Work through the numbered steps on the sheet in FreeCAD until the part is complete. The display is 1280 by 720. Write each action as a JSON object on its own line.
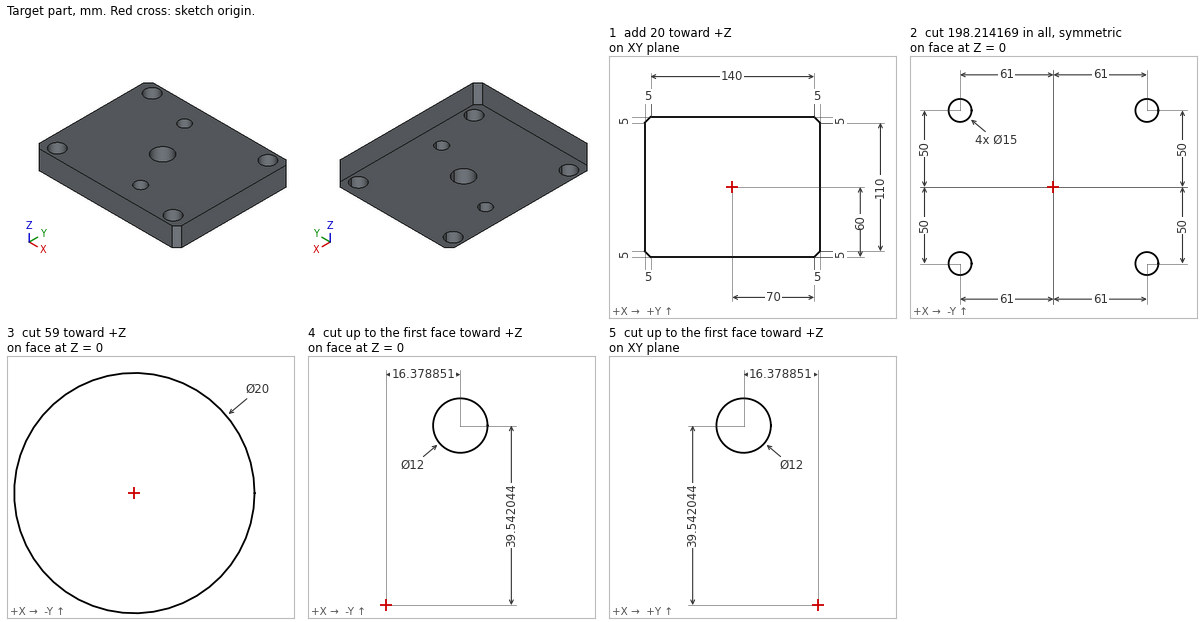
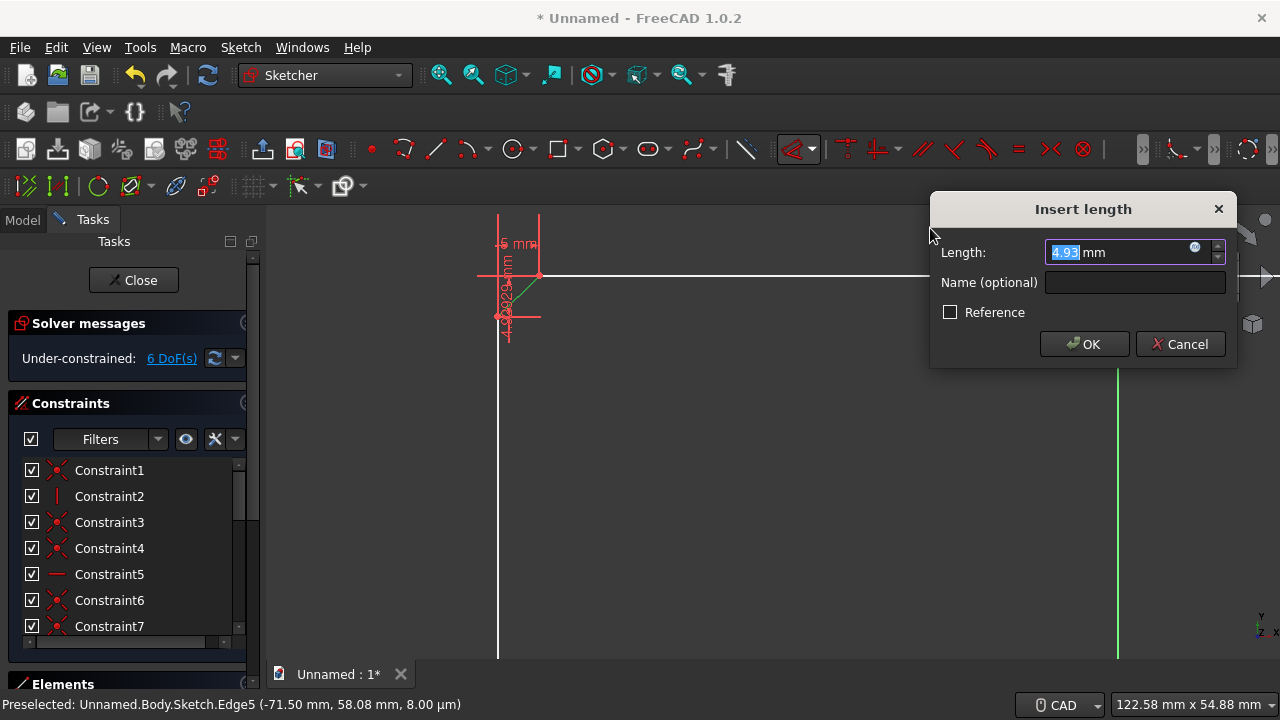
{"action": "type", "text": "5"}
{"action": "key", "text": "Return"}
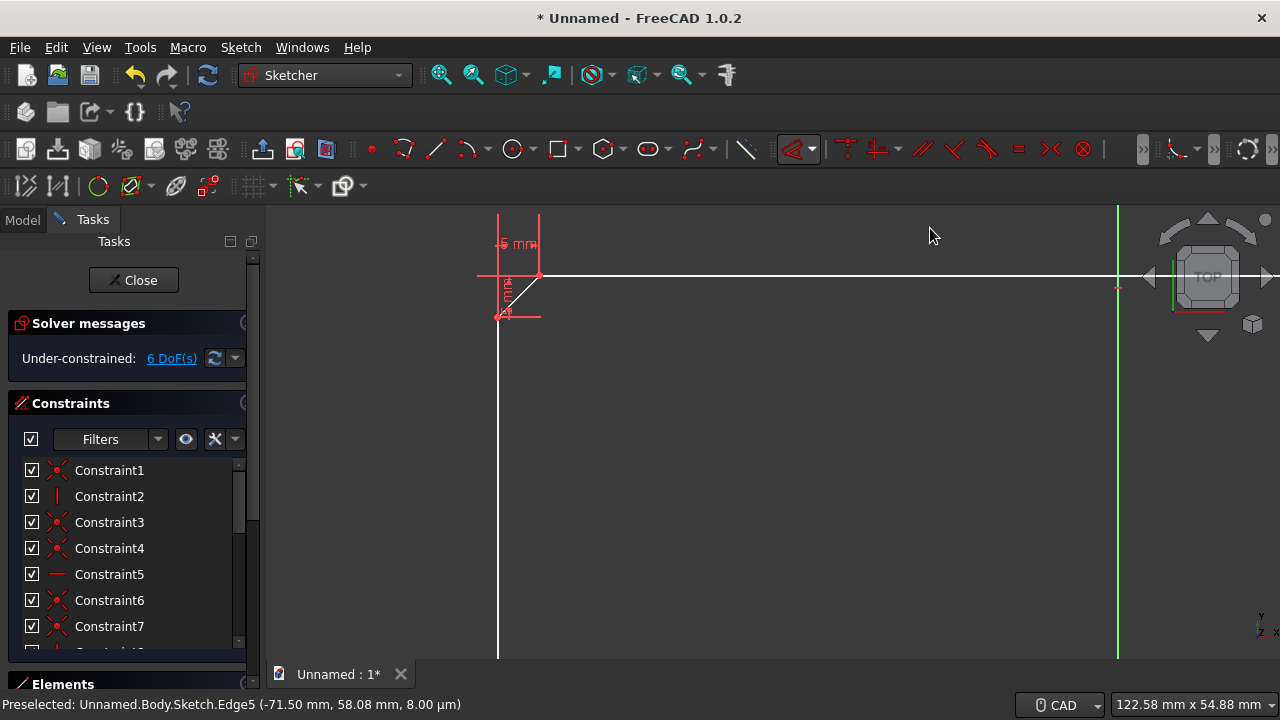
{"action": "scroll", "coordinate": [526, 287], "scroll_direction": "down", "scroll_amount": 6}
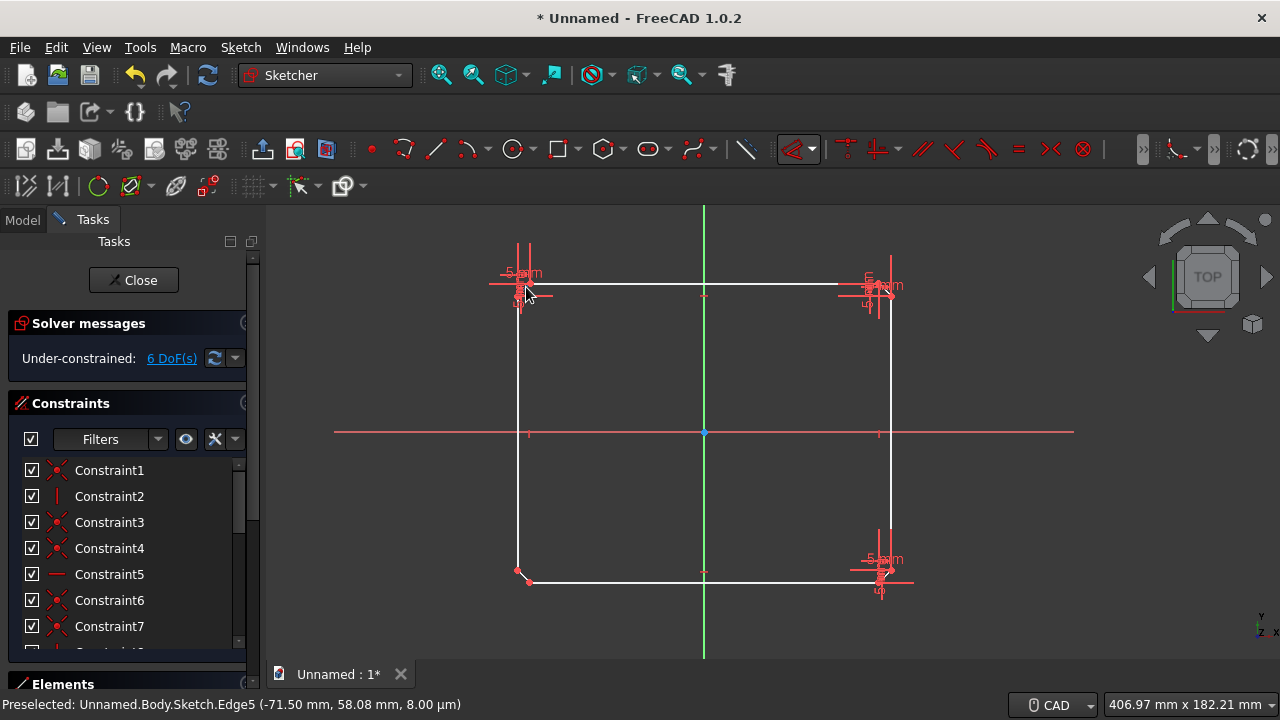
{"action": "scroll", "coordinate": [521, 574], "scroll_direction": "up", "scroll_amount": 6}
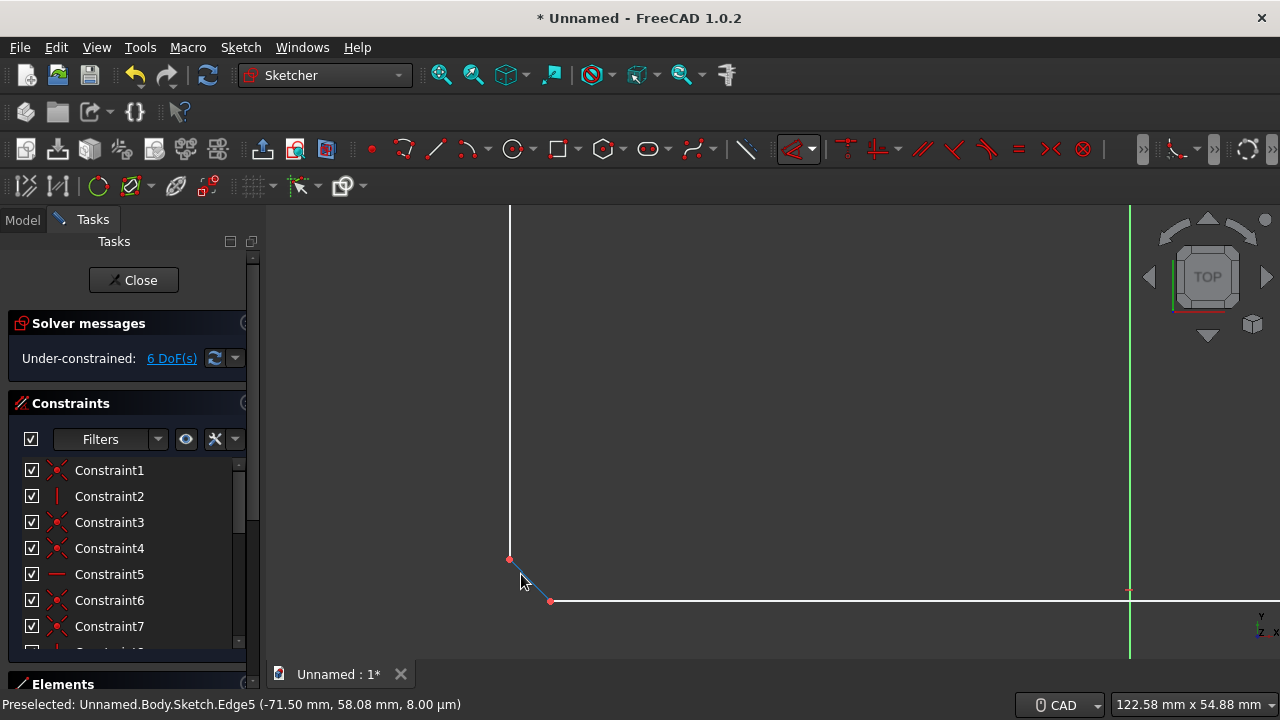
{"action": "left_click", "coordinate": [522, 572]}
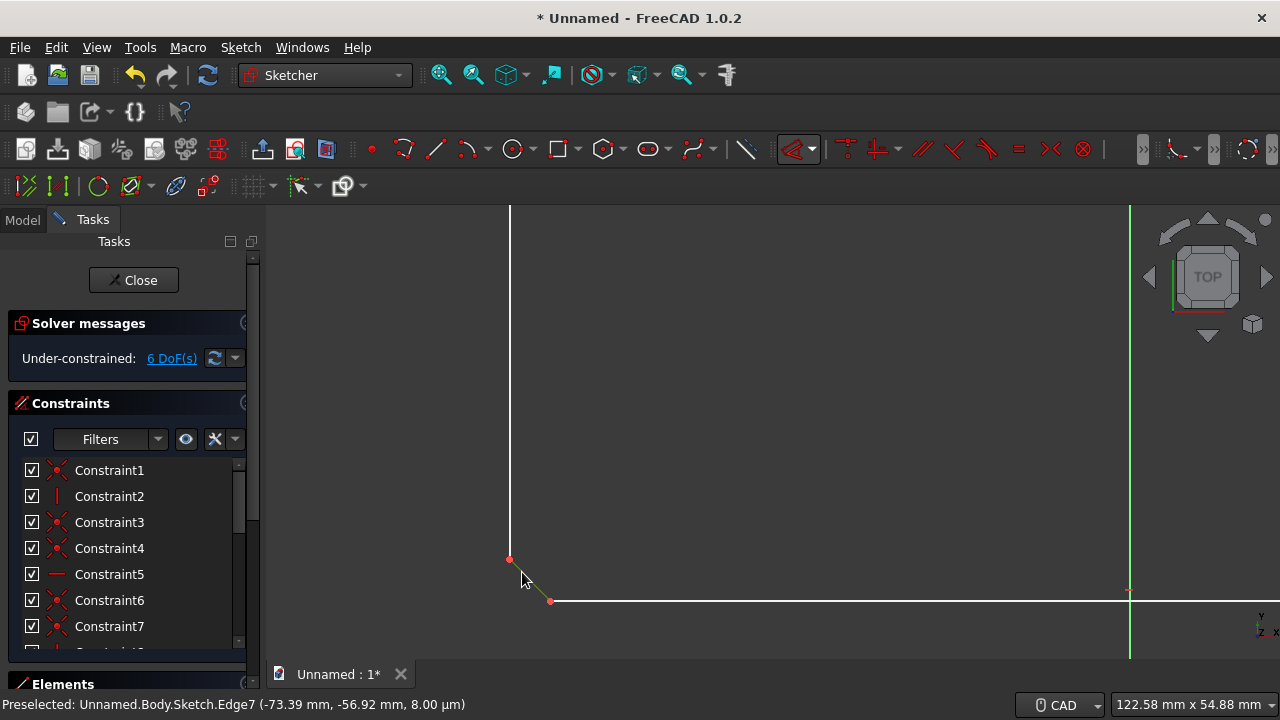
{"action": "left_click", "coordinate": [814, 150]}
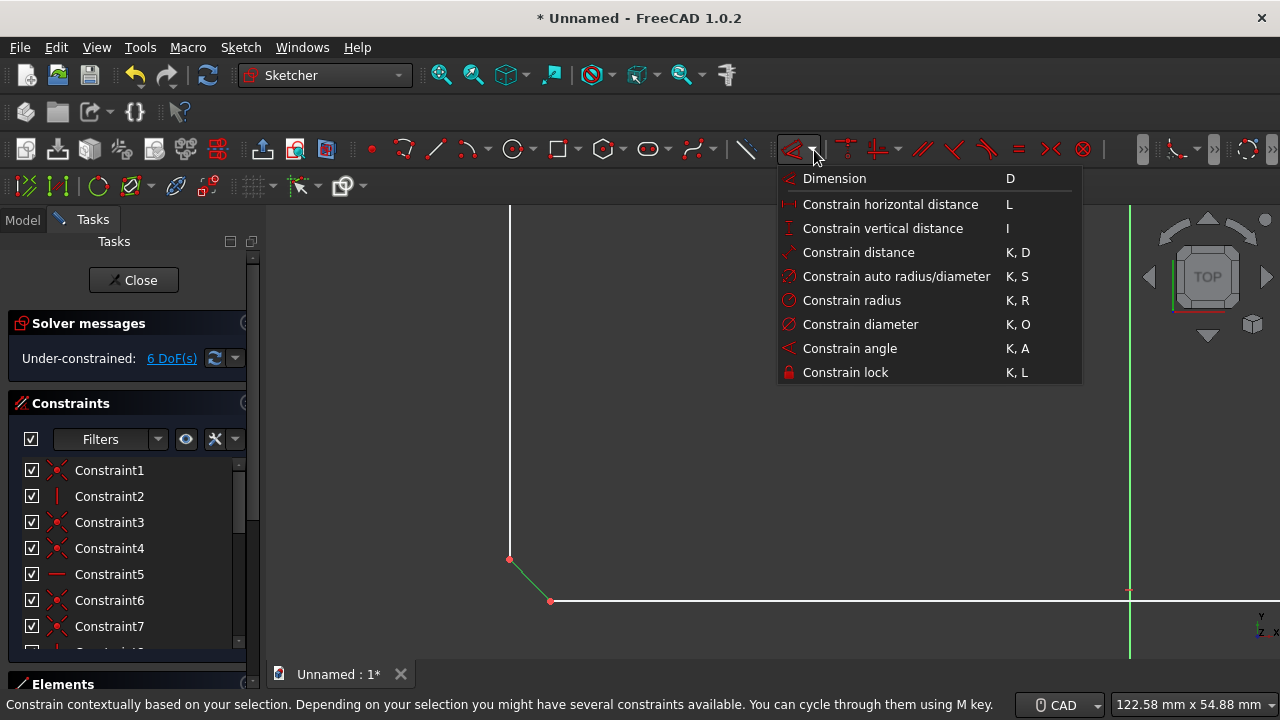
{"action": "left_click", "coordinate": [930, 204]}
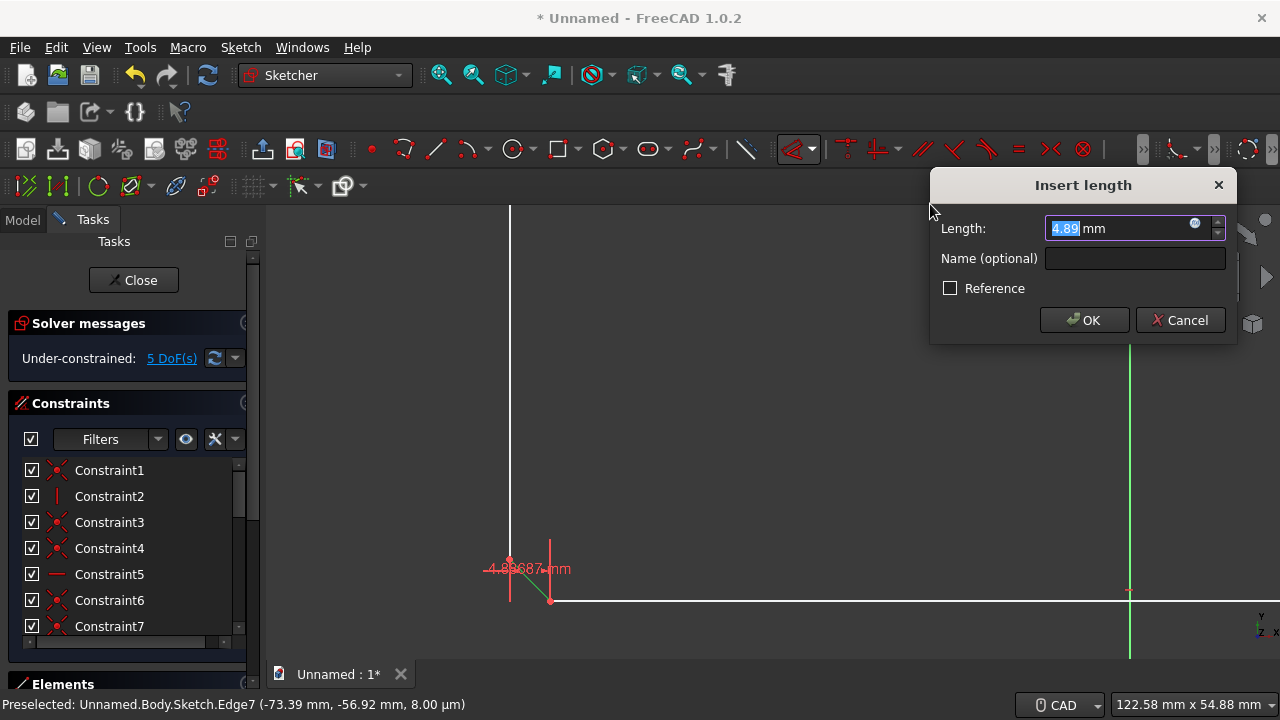
{"action": "type", "text": "5"}
{"action": "key", "text": "Return"}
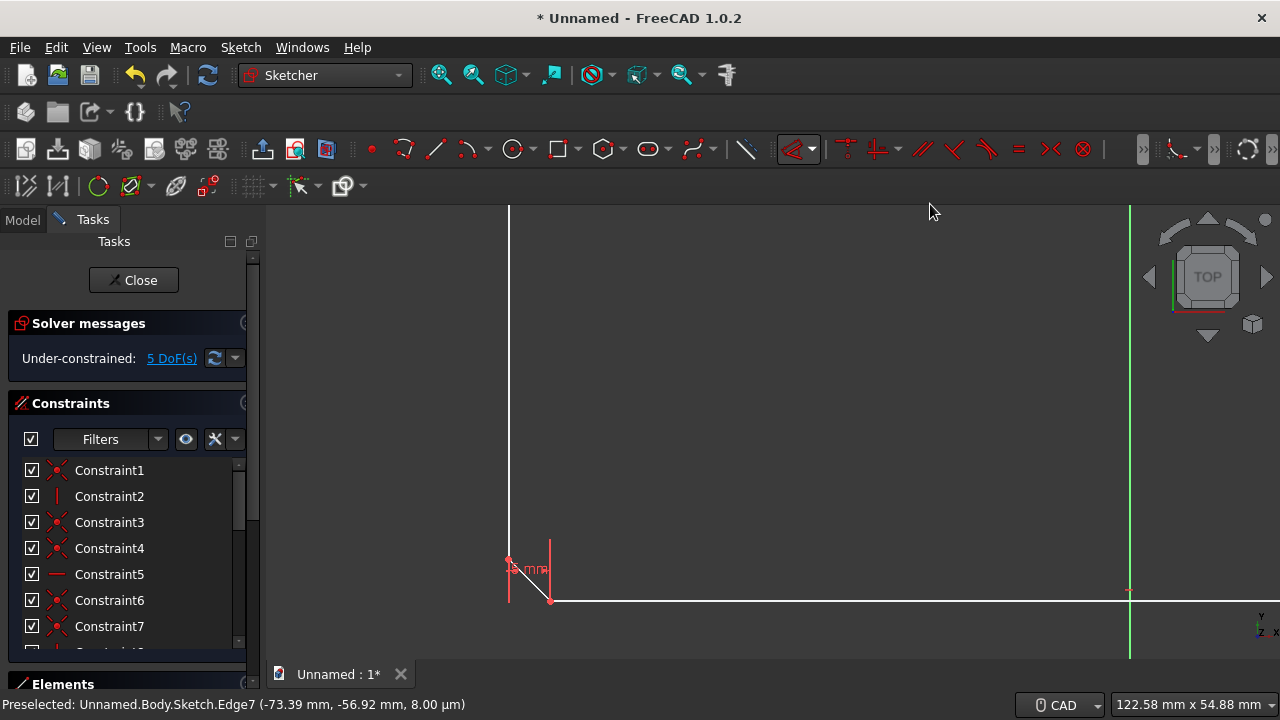
{"action": "left_click", "coordinate": [538, 588]}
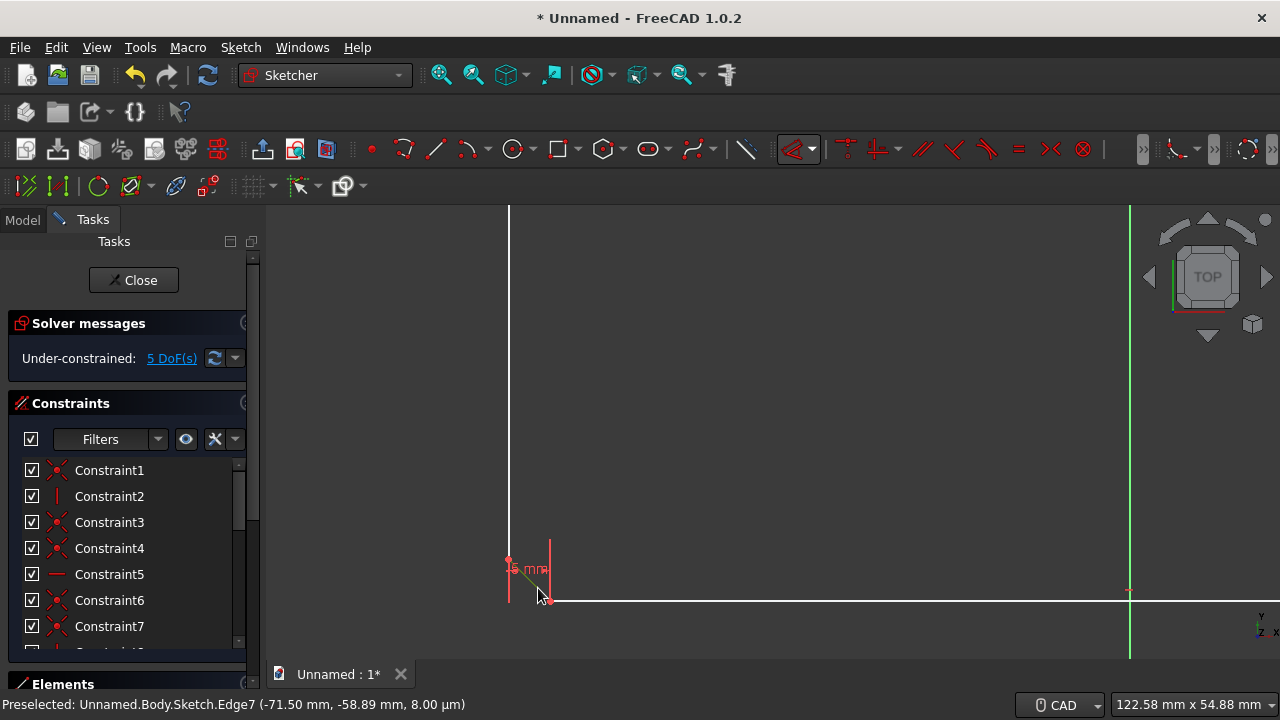
{"action": "left_click", "coordinate": [814, 150]}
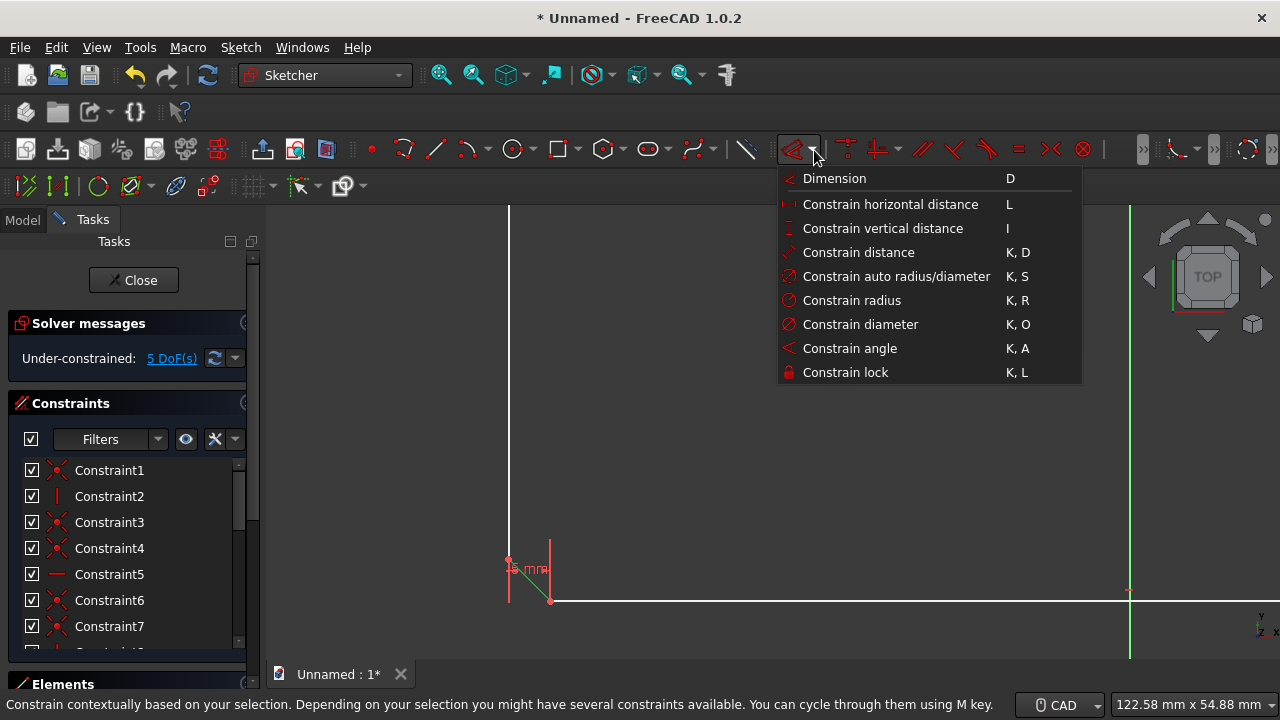
{"action": "left_click", "coordinate": [930, 228]}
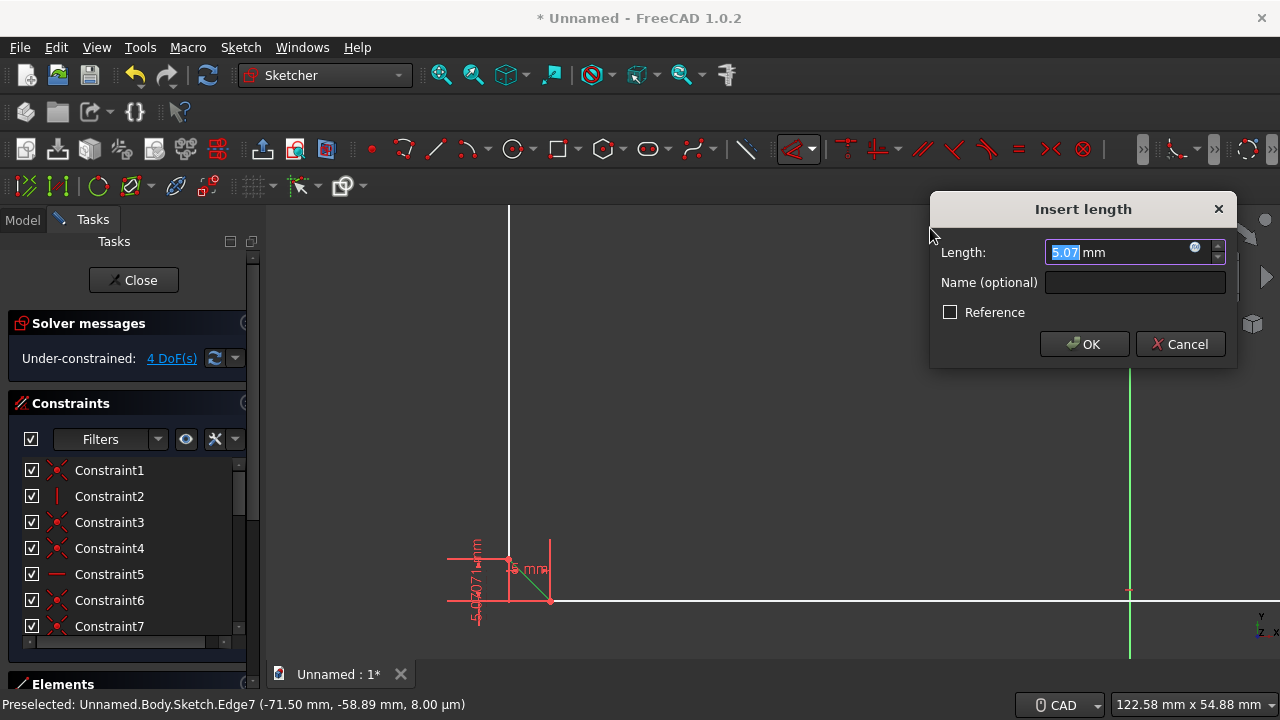
{"action": "type", "text": "5"}
{"action": "key", "text": "Return"}